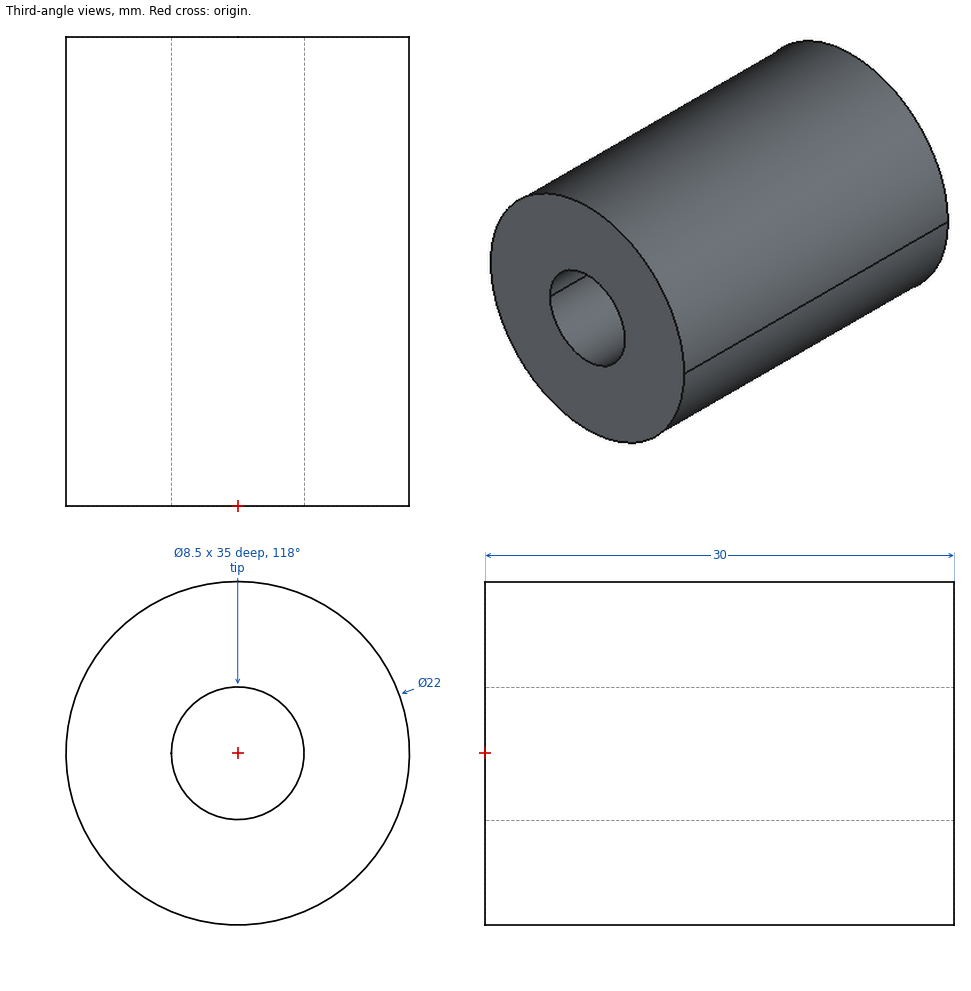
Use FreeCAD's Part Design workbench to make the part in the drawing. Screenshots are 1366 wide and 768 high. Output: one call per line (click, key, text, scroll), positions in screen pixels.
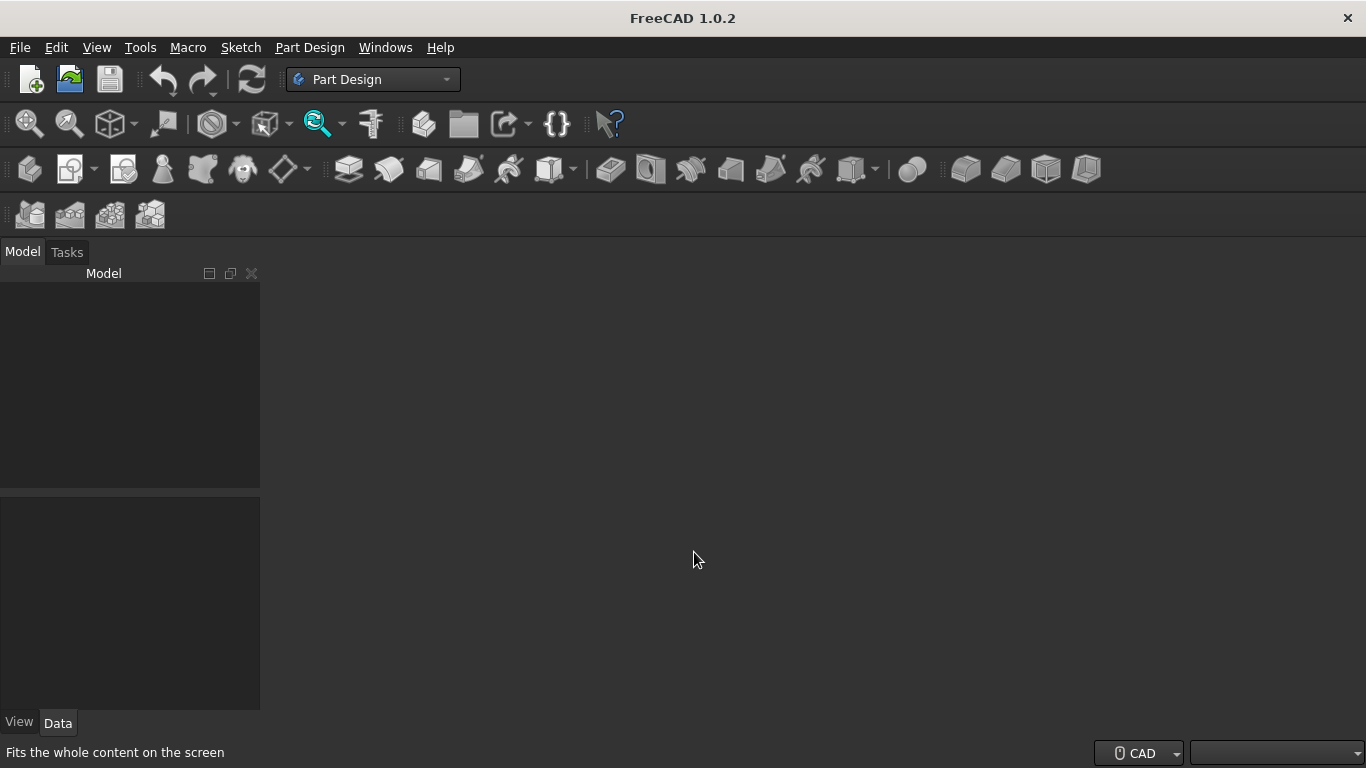
click(30, 80)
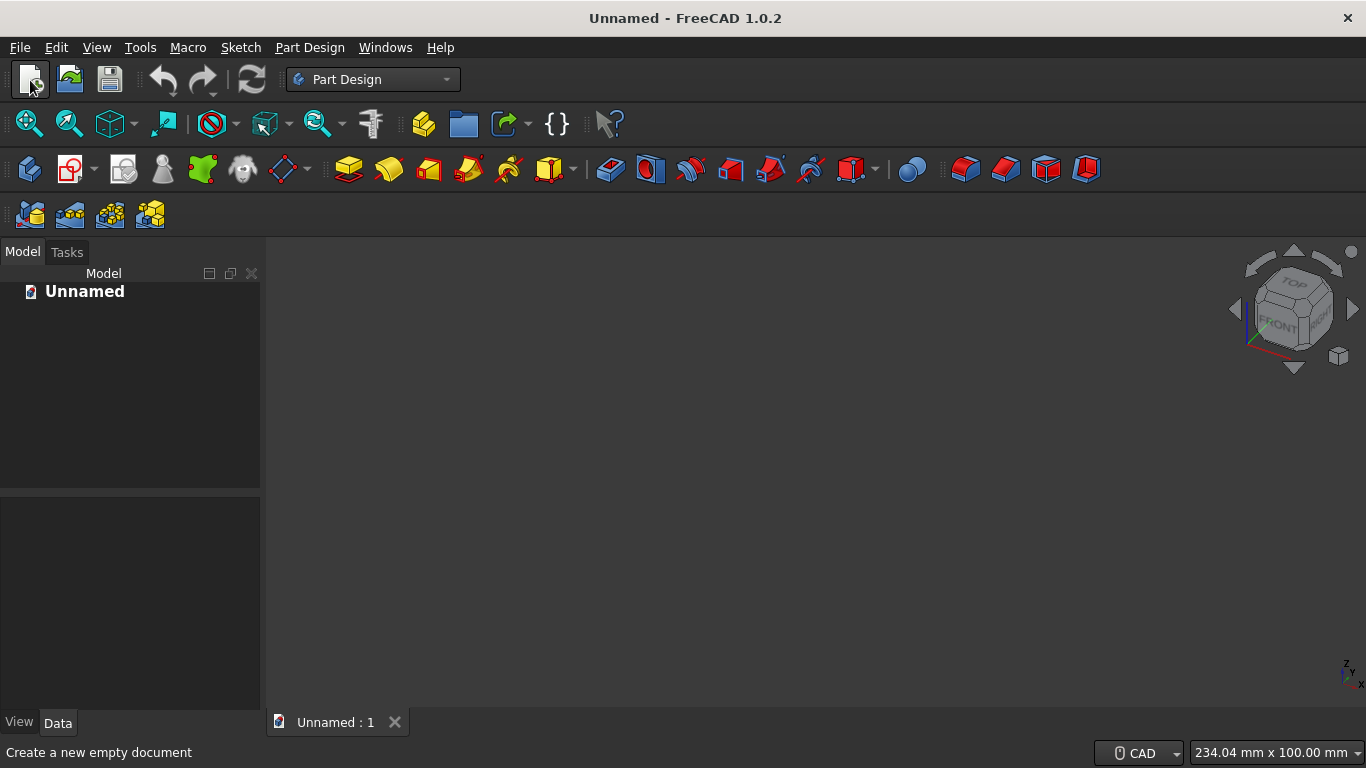
click(70, 170)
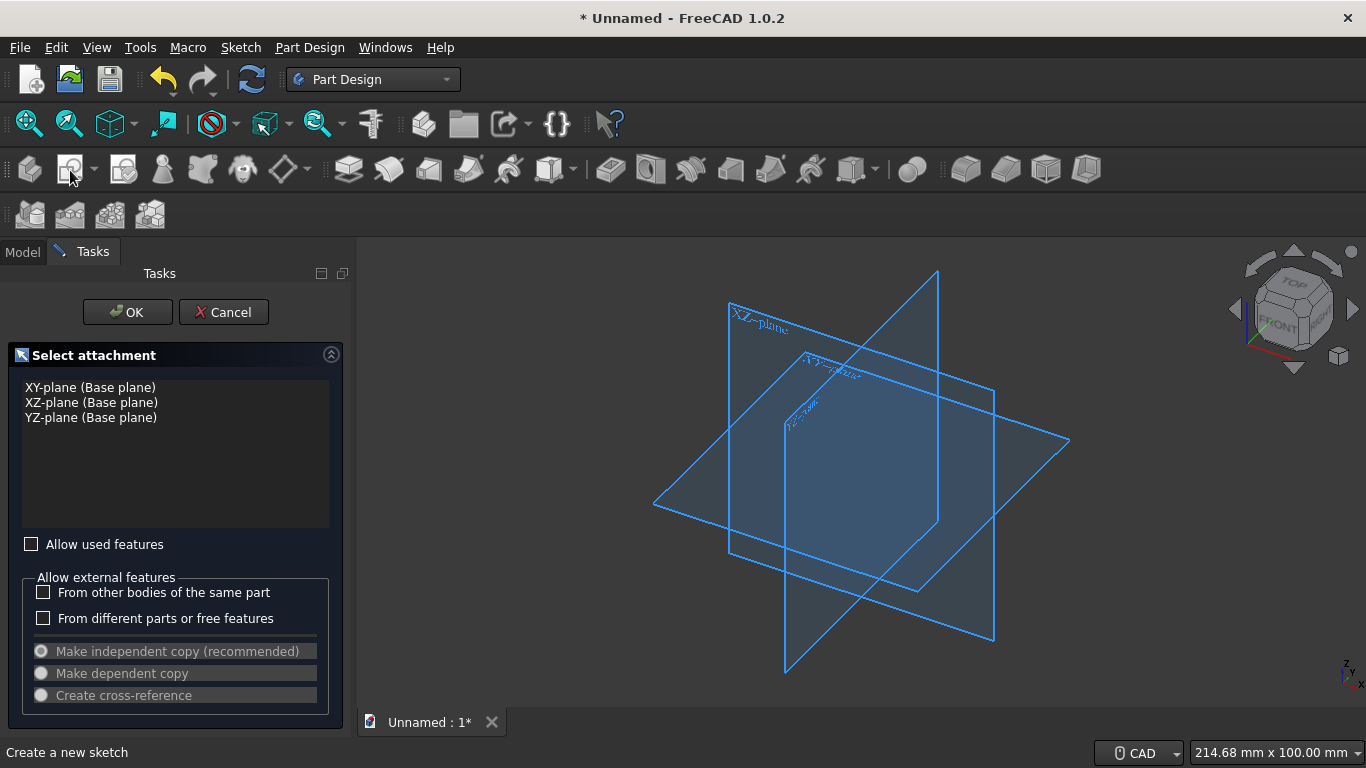
click(82, 402)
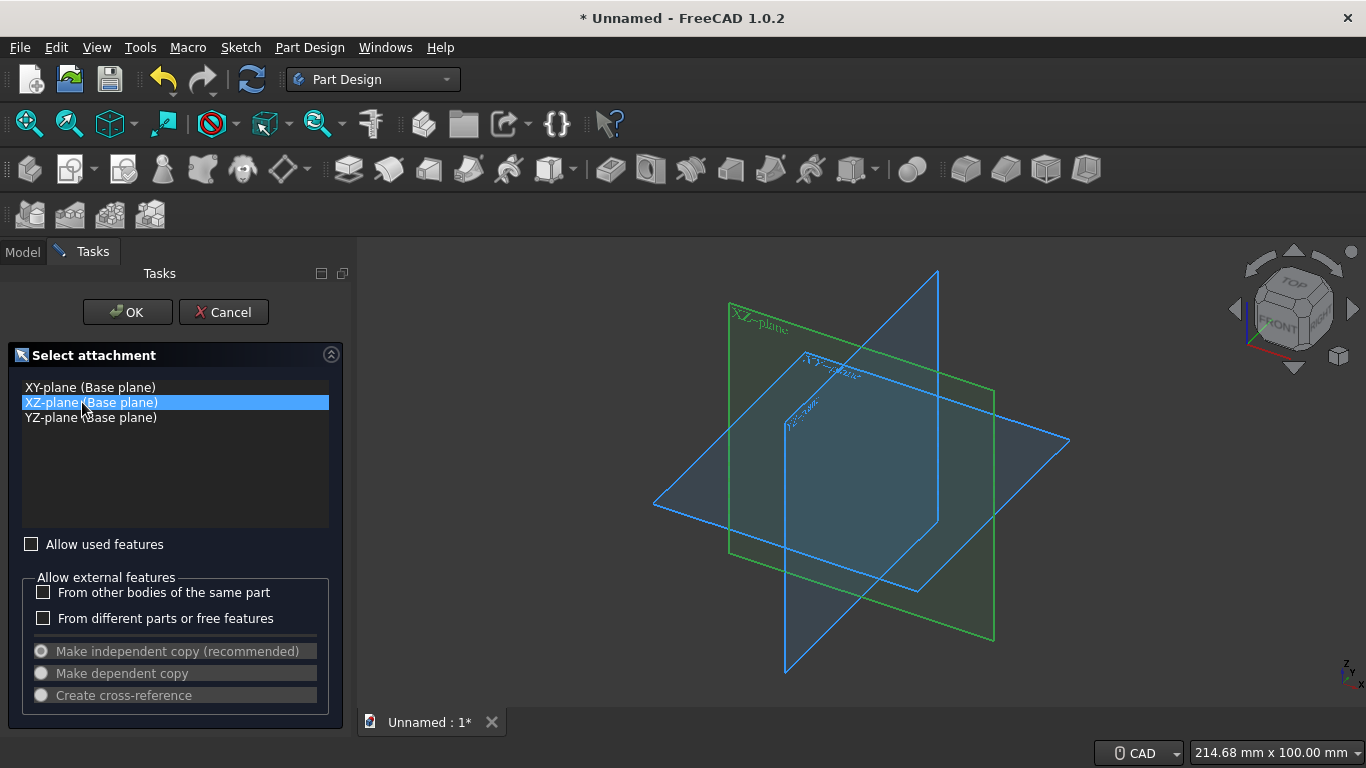
click(128, 312)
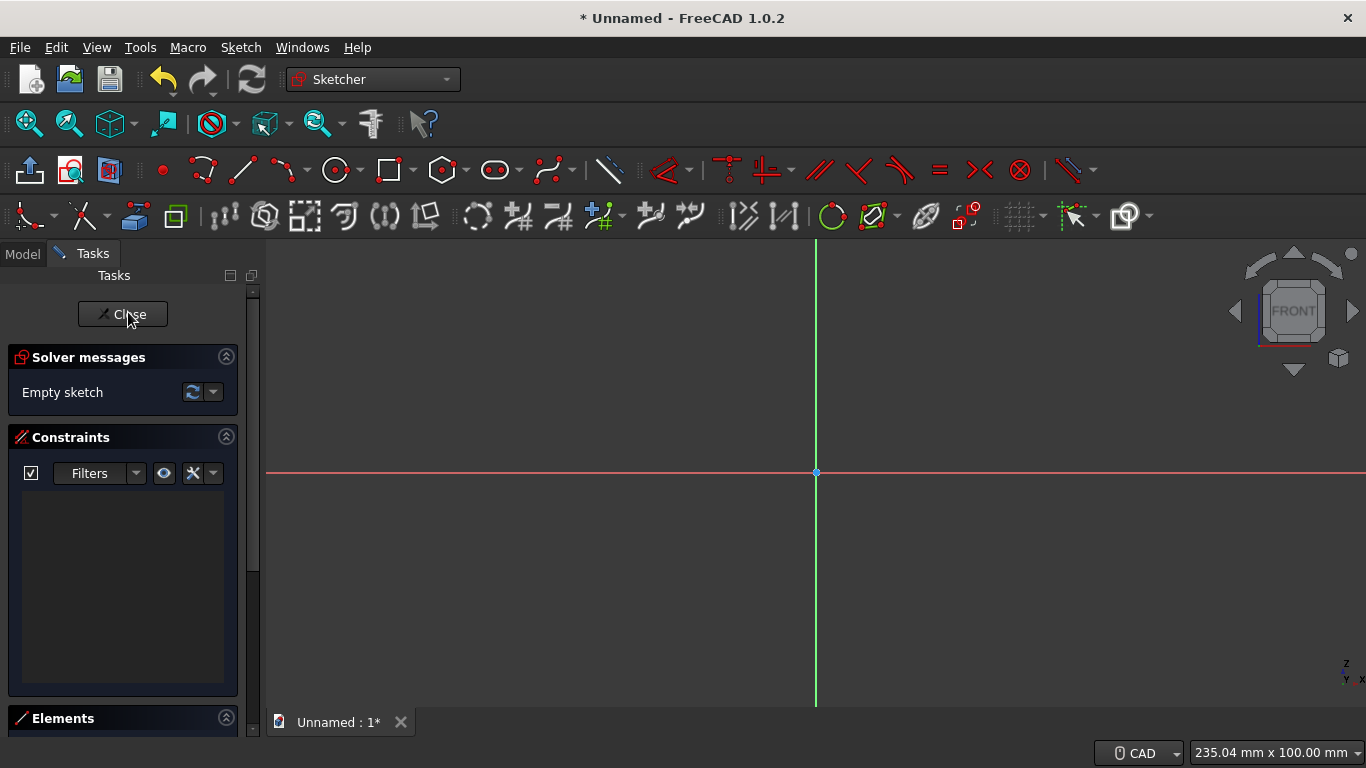
scroll(856, 473, up, 5)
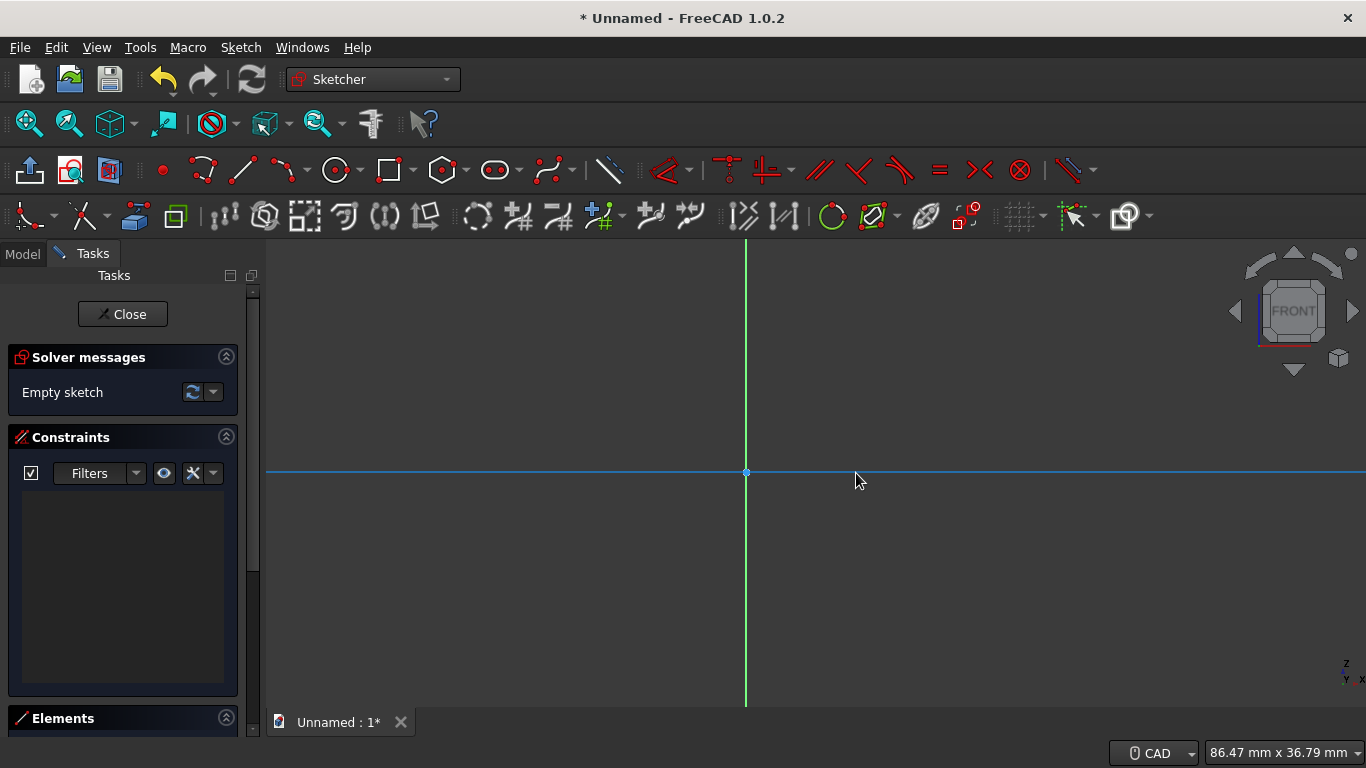
click(336, 170)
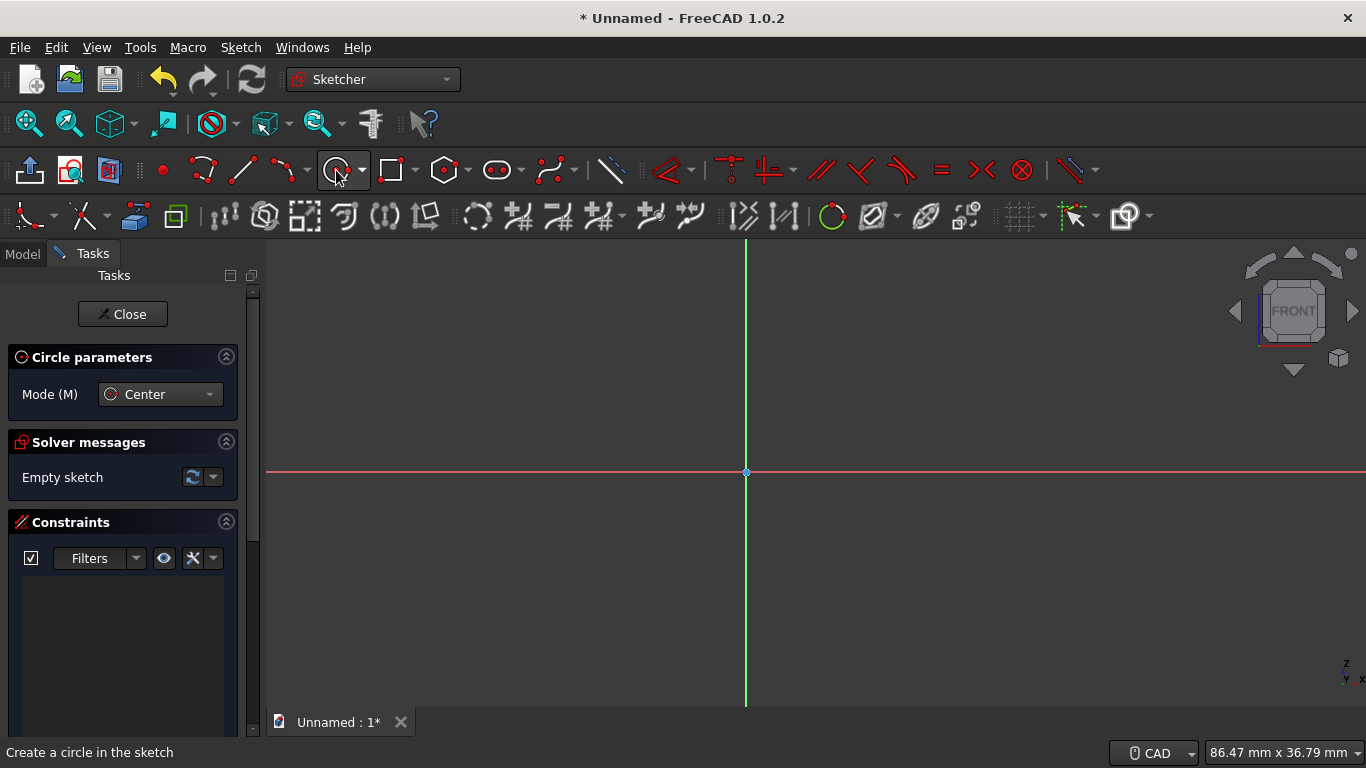
click(746, 472)
click(845, 373)
key(Escape)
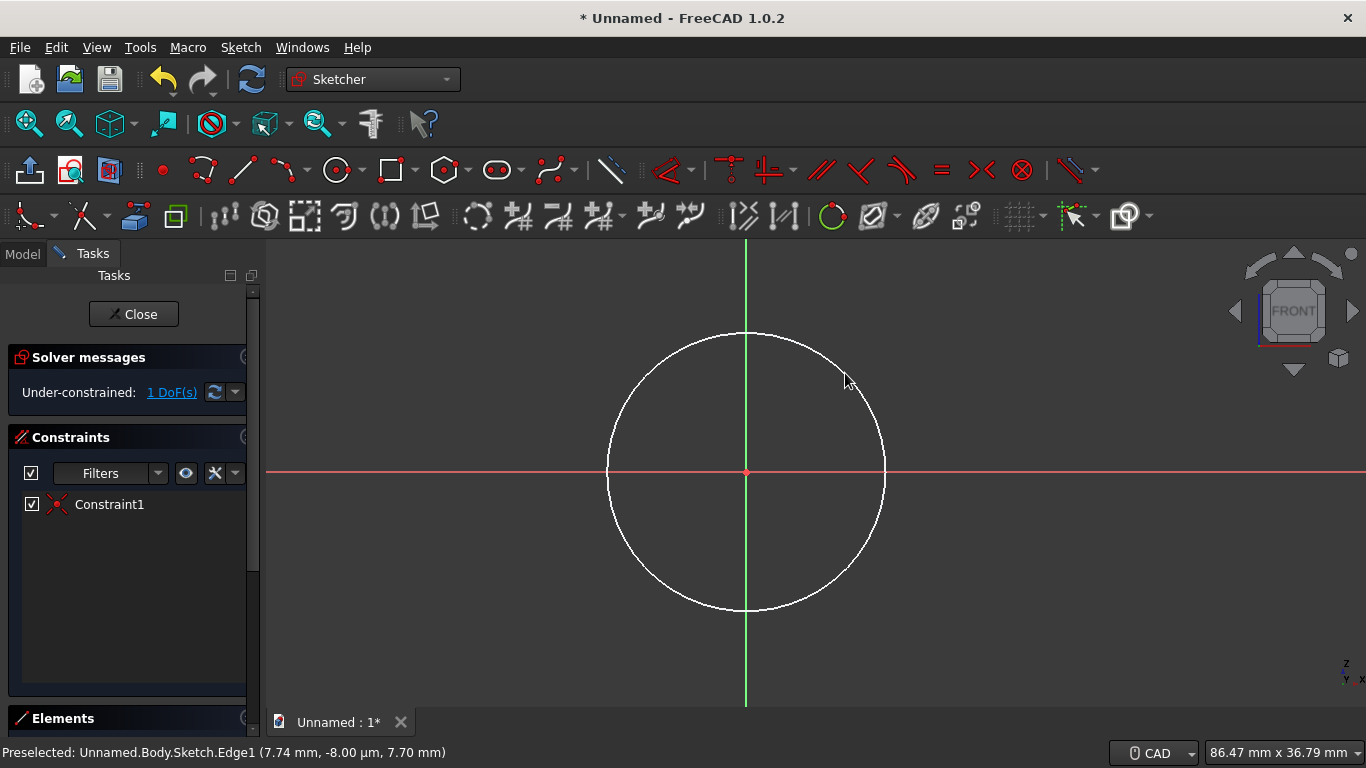
click(666, 170)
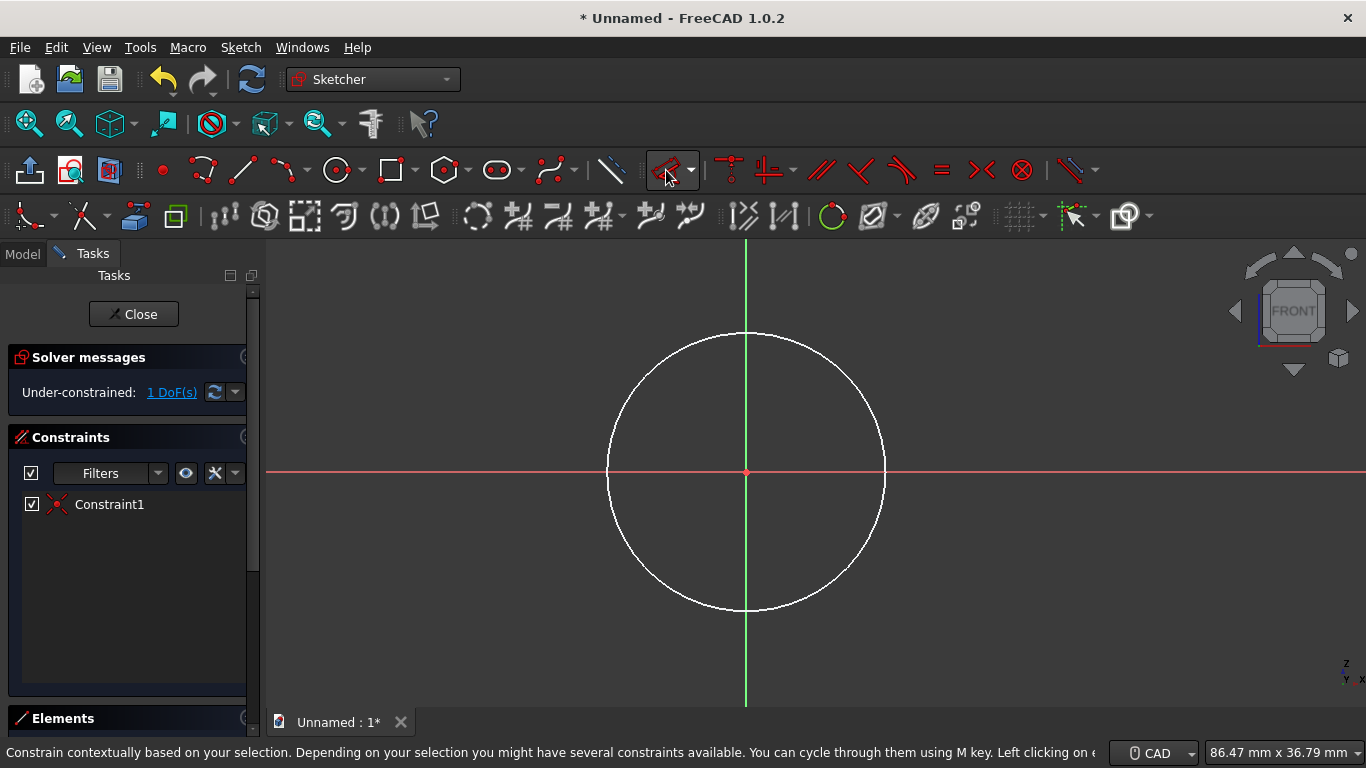
click(844, 373)
click(866, 350)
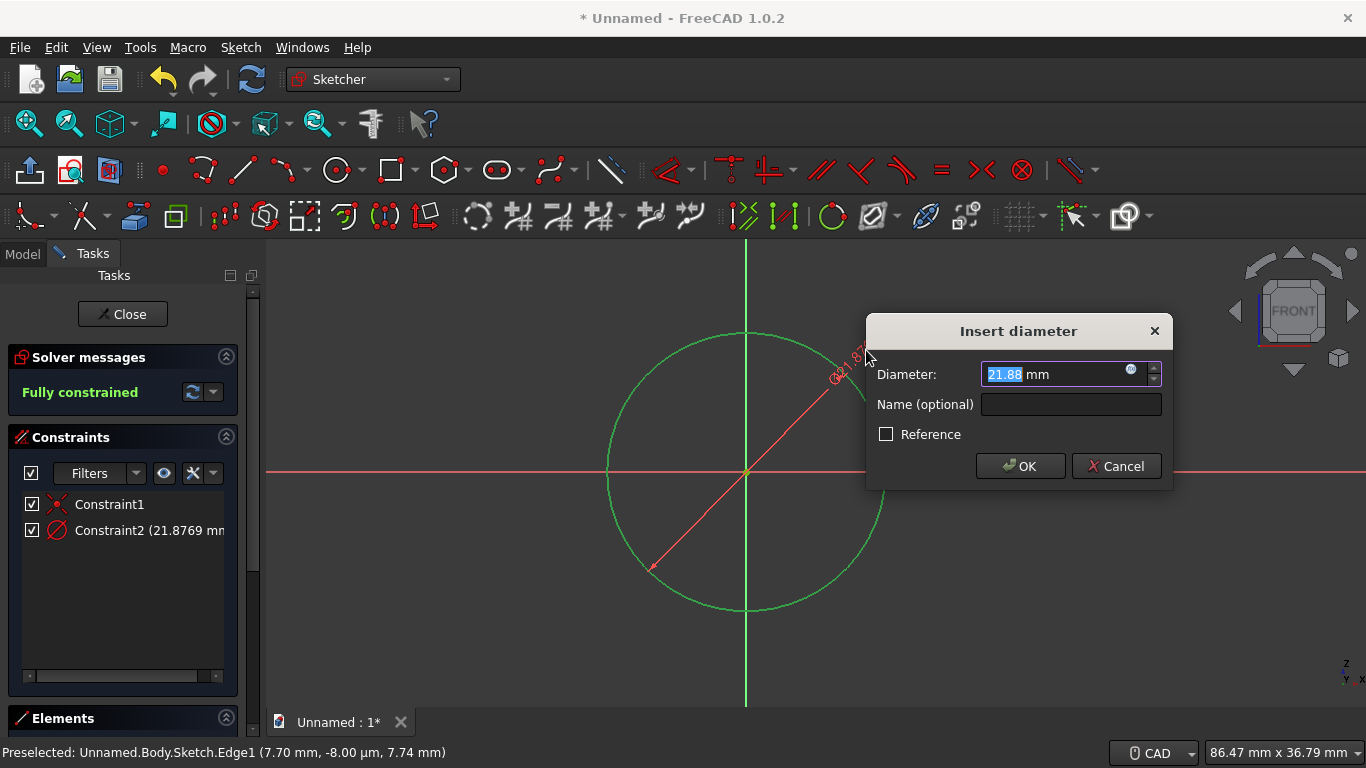
text(22)
key(Return)
key(Escape)